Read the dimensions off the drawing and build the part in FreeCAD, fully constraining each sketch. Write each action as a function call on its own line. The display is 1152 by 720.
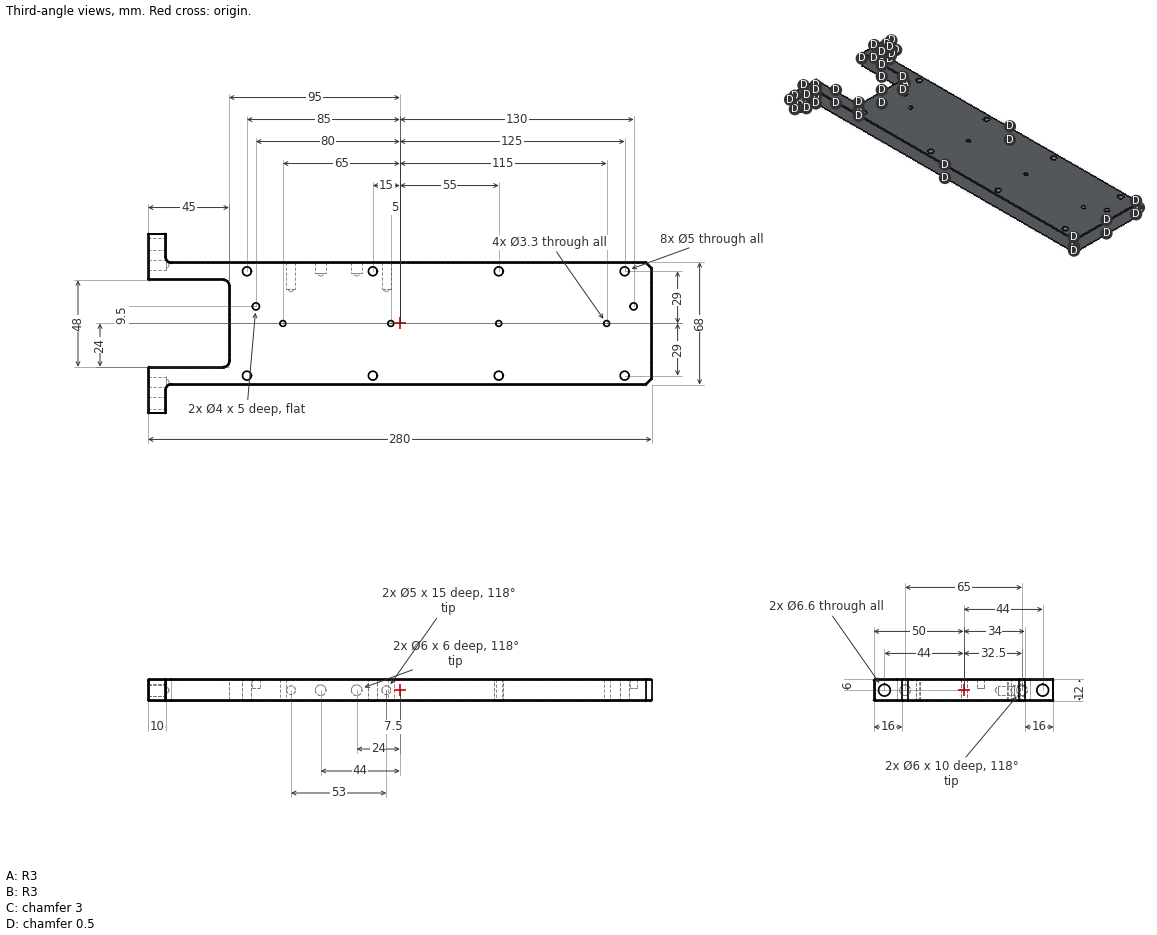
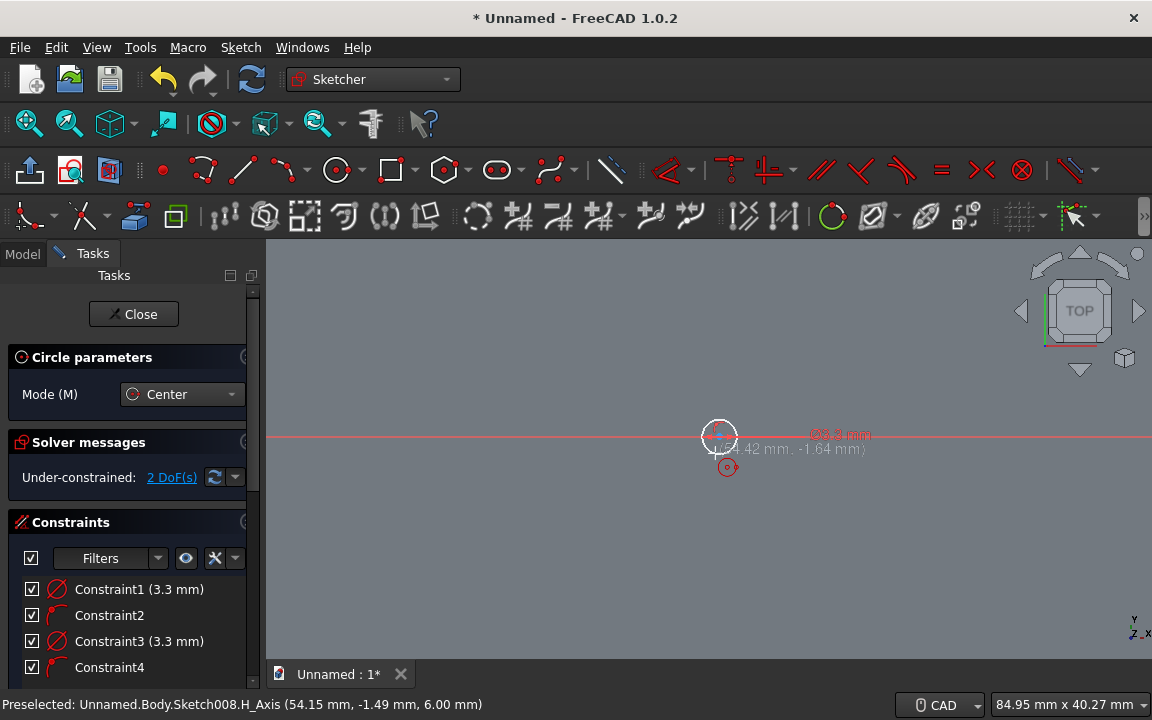
scroll(717, 453, down, 7)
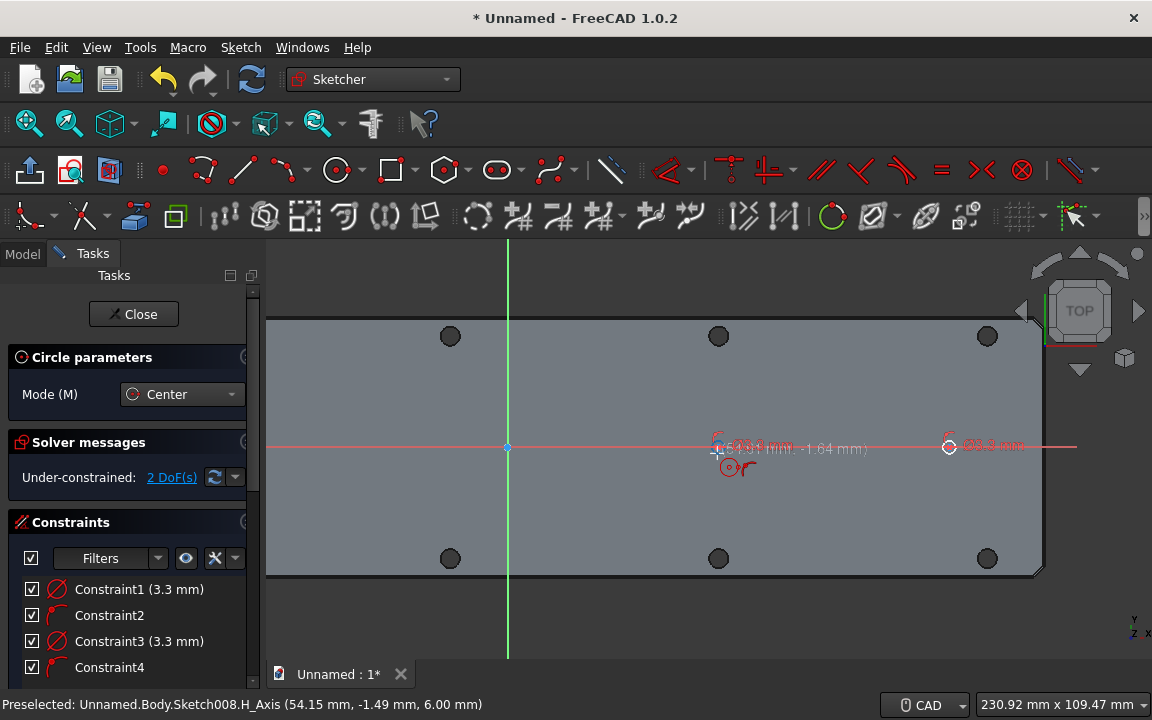
scroll(410, 449, up, 9)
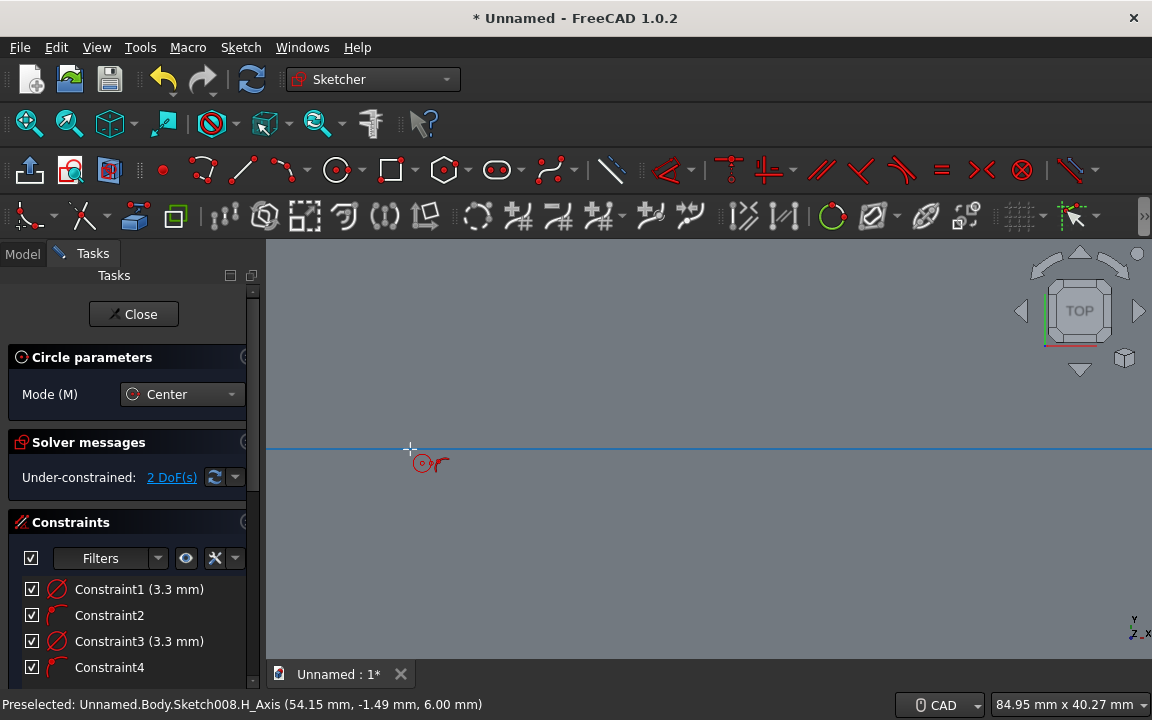
scroll(409, 449, down, 9)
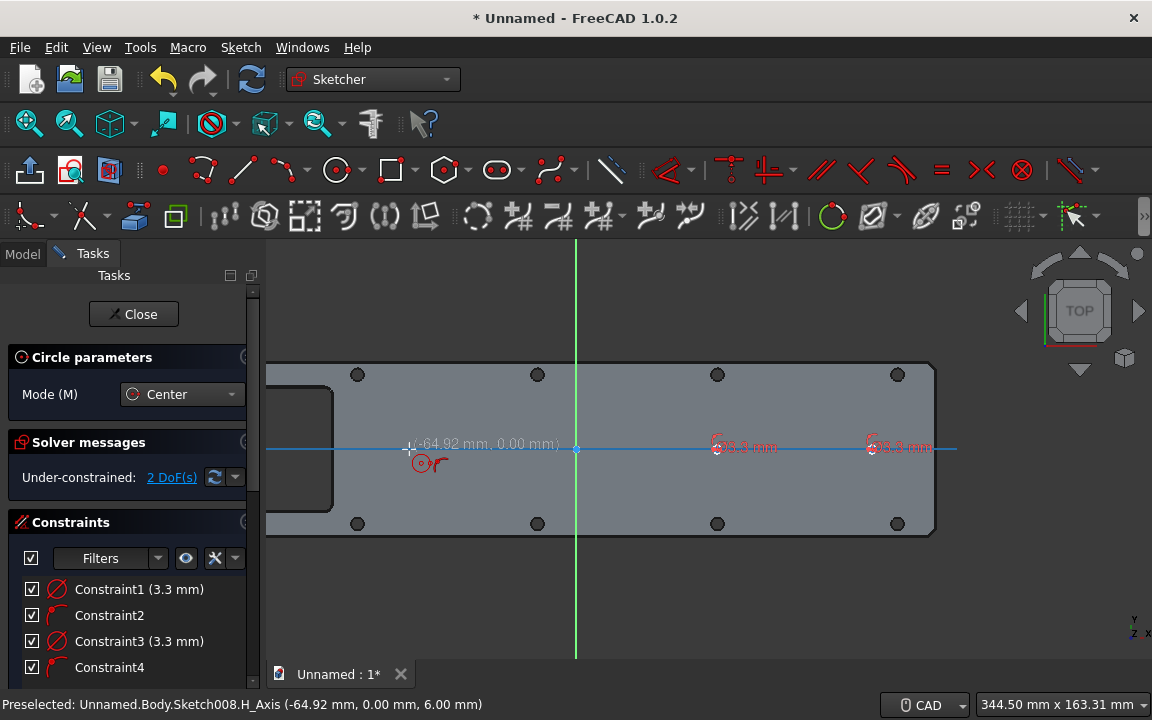
click(409, 449)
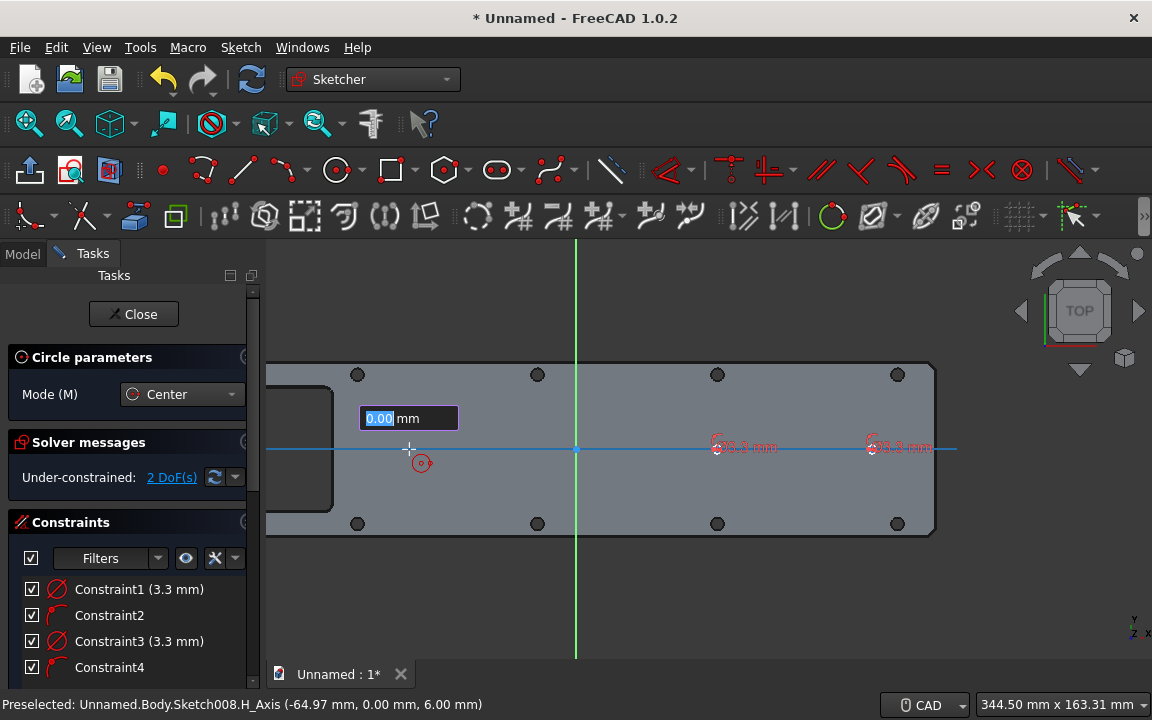
scroll(407, 453, up, 7)
move(408, 453)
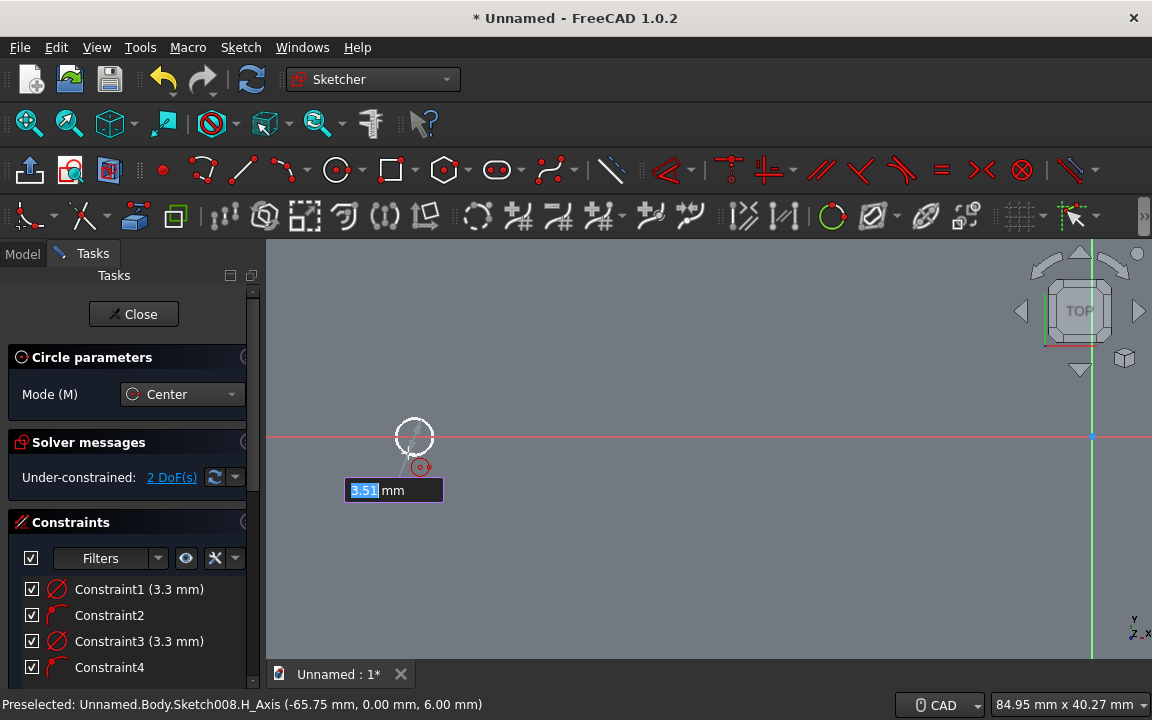
text(3.3)
key(Return)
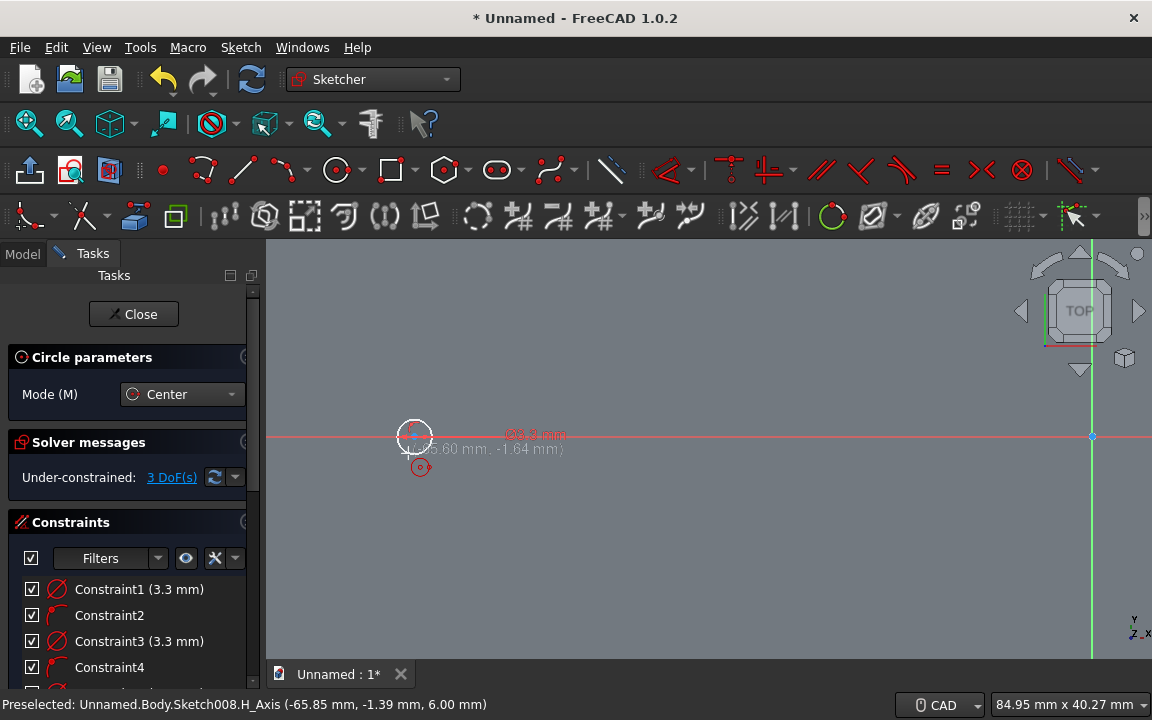
scroll(407, 453, down, 7)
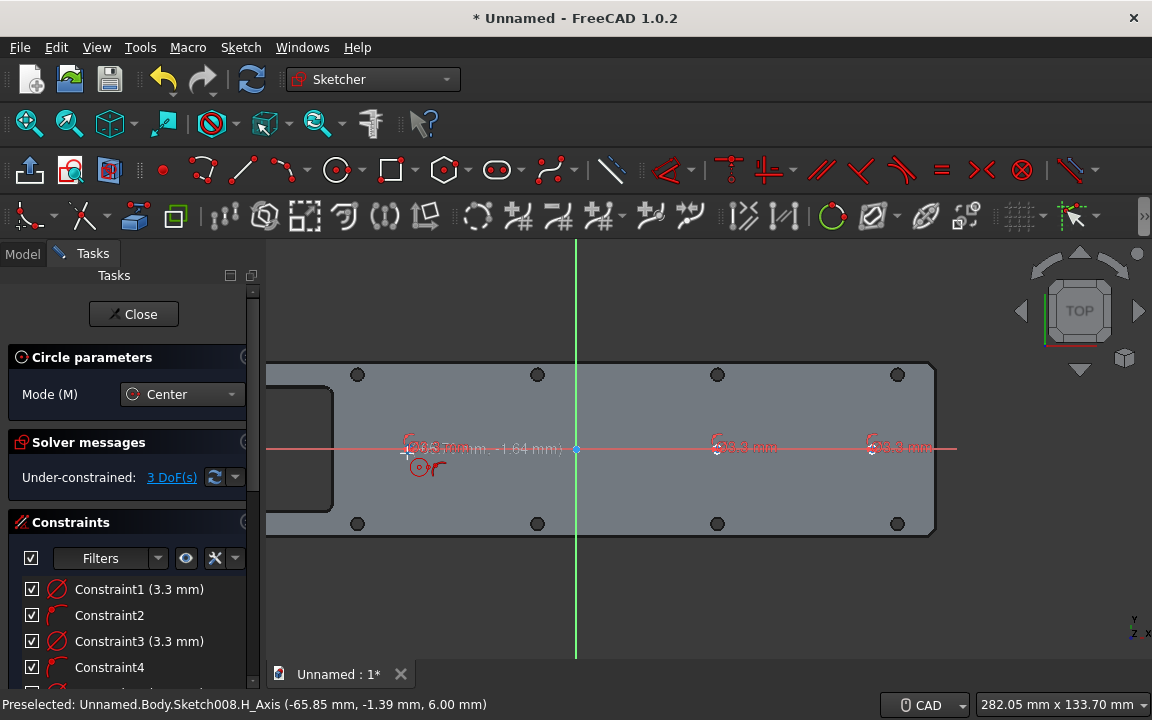
scroll(563, 449, up, 9)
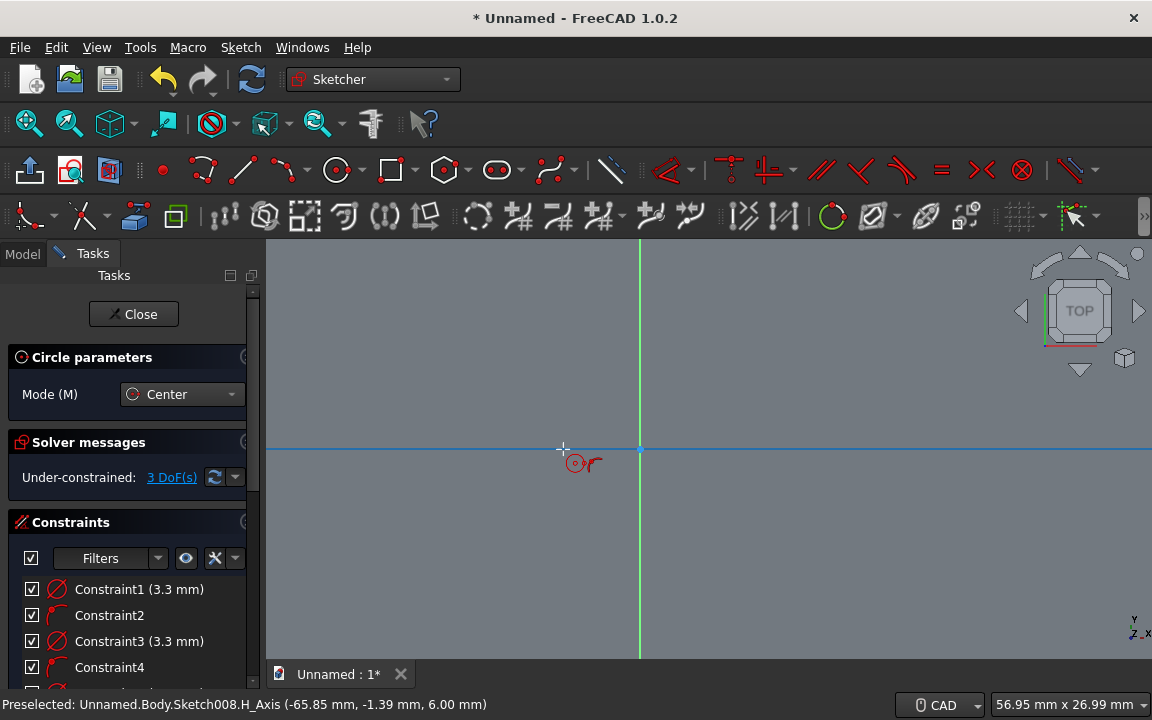
scroll(563, 449, down, 9)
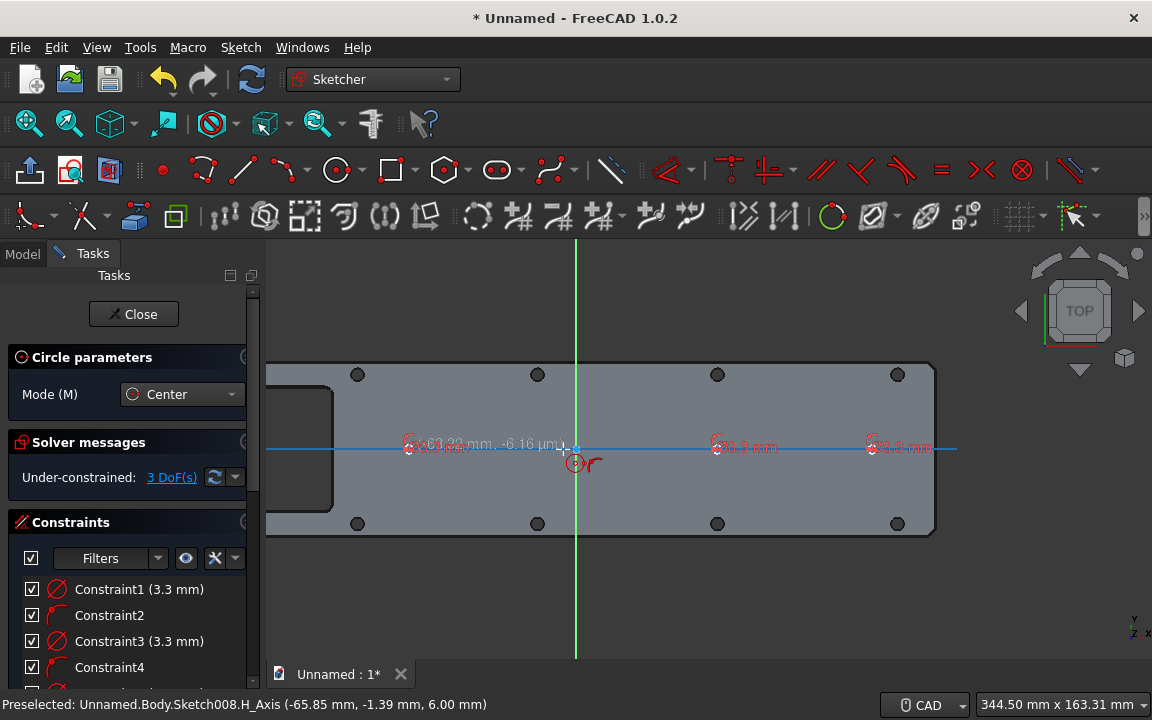
scroll(563, 449, up, 2)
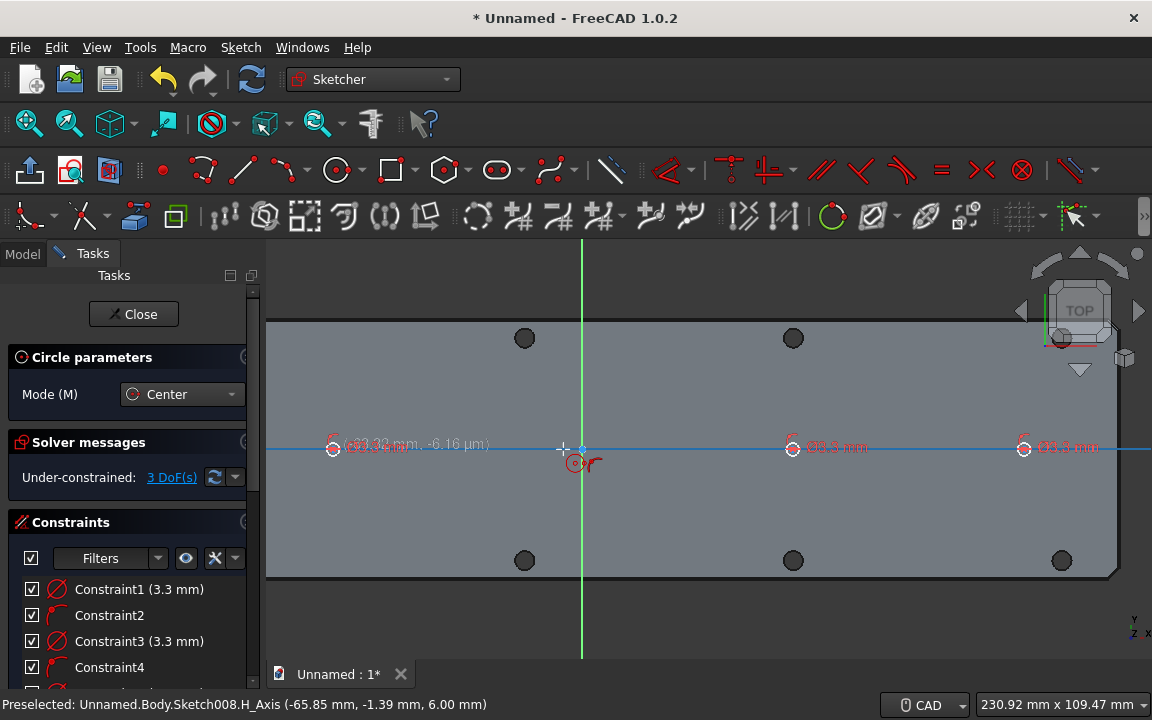
click(563, 449)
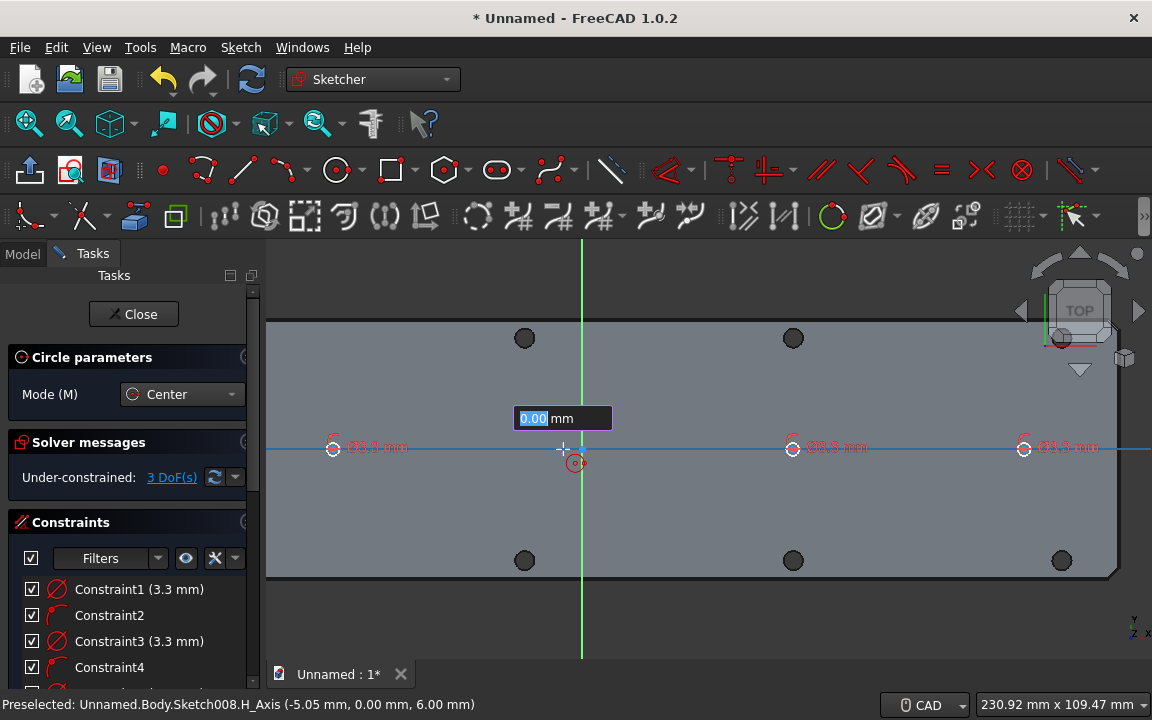
scroll(561, 455, up, 5)
move(560, 455)